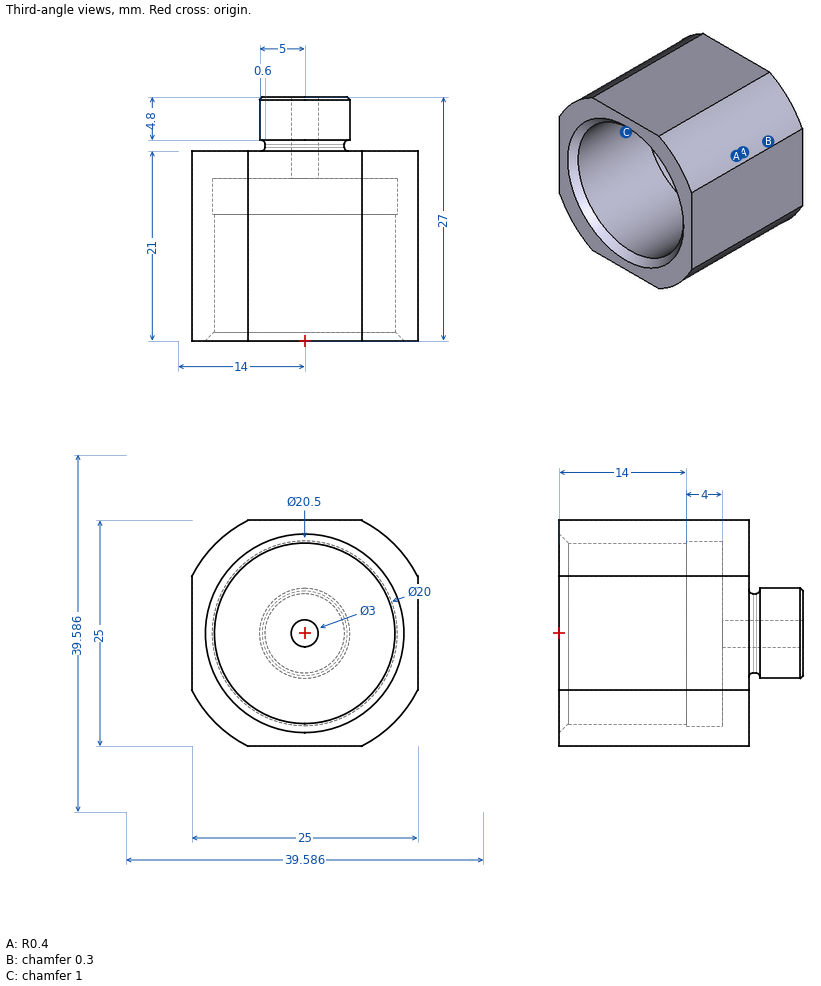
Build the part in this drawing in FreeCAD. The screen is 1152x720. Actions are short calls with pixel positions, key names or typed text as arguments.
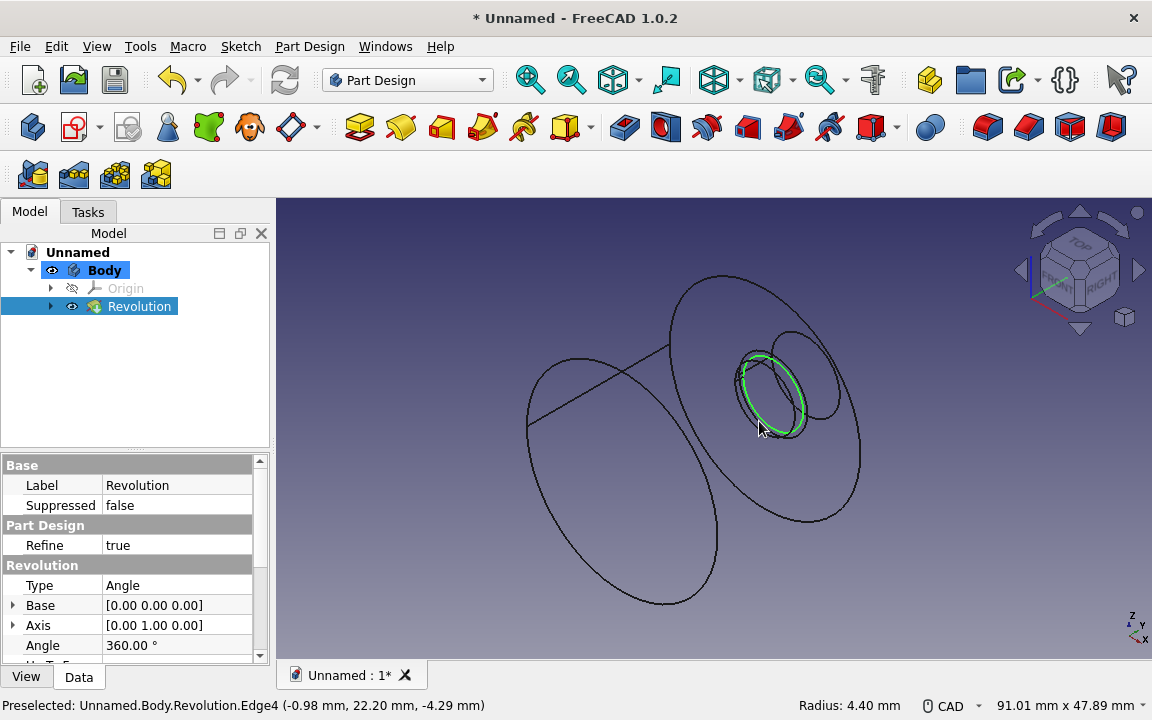
click(795, 415, ctrl)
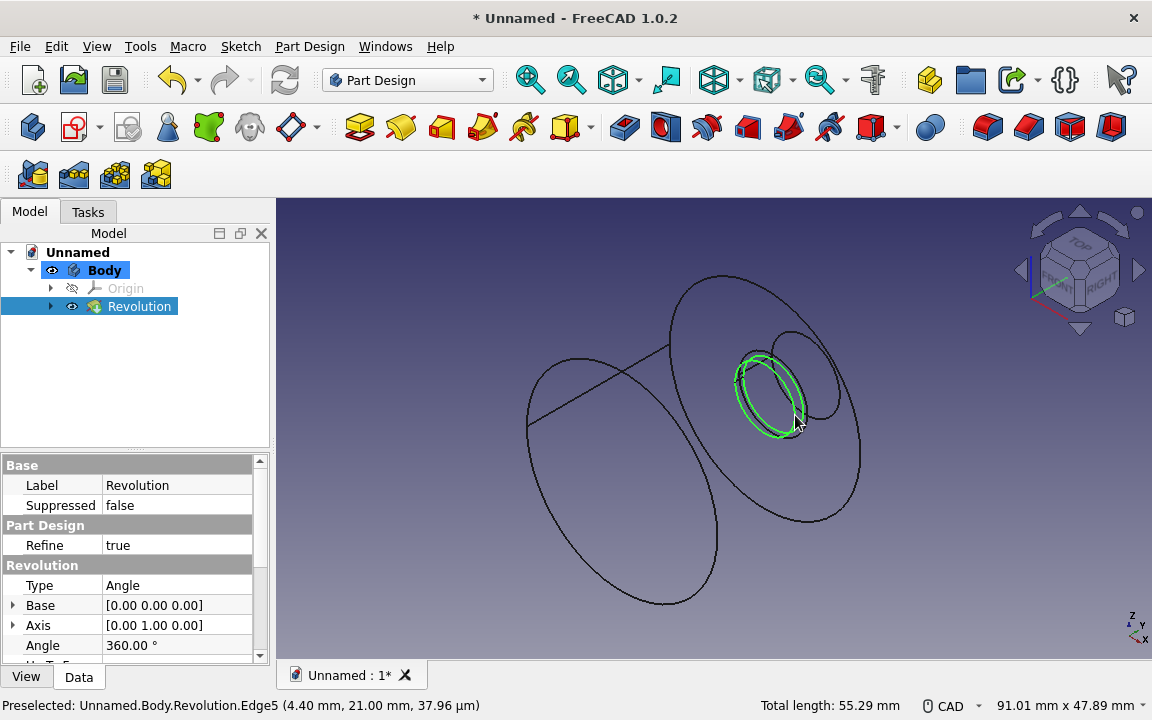
key(v)
key(1)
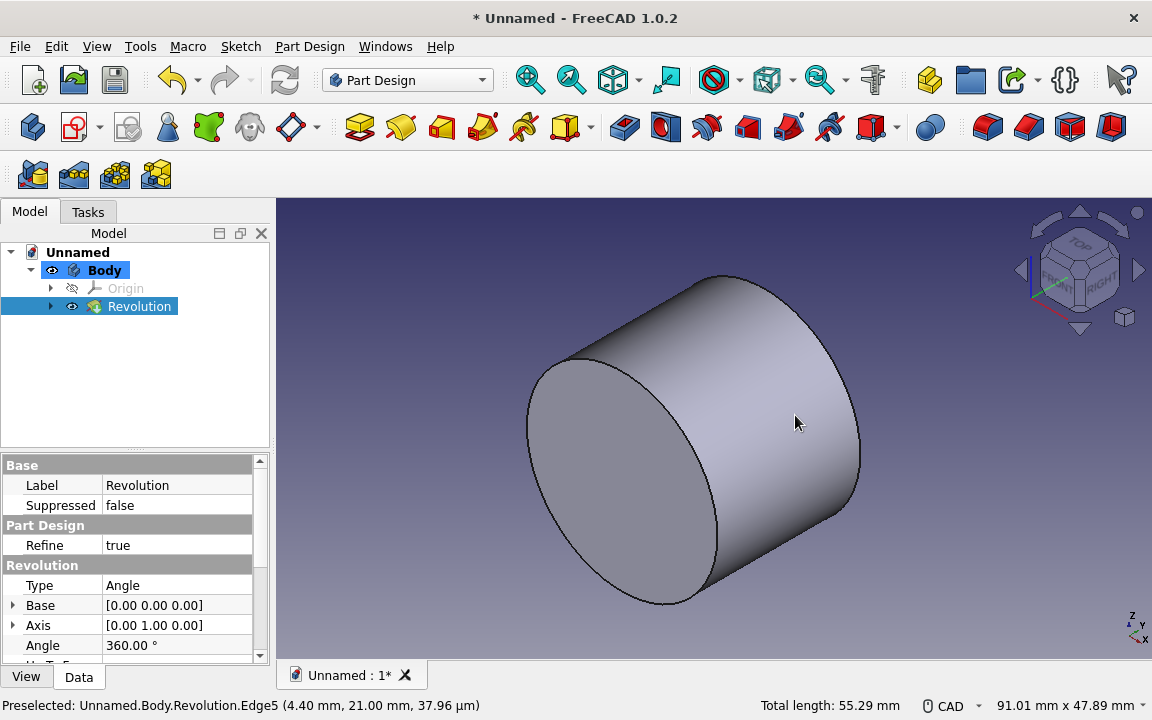
click(988, 128)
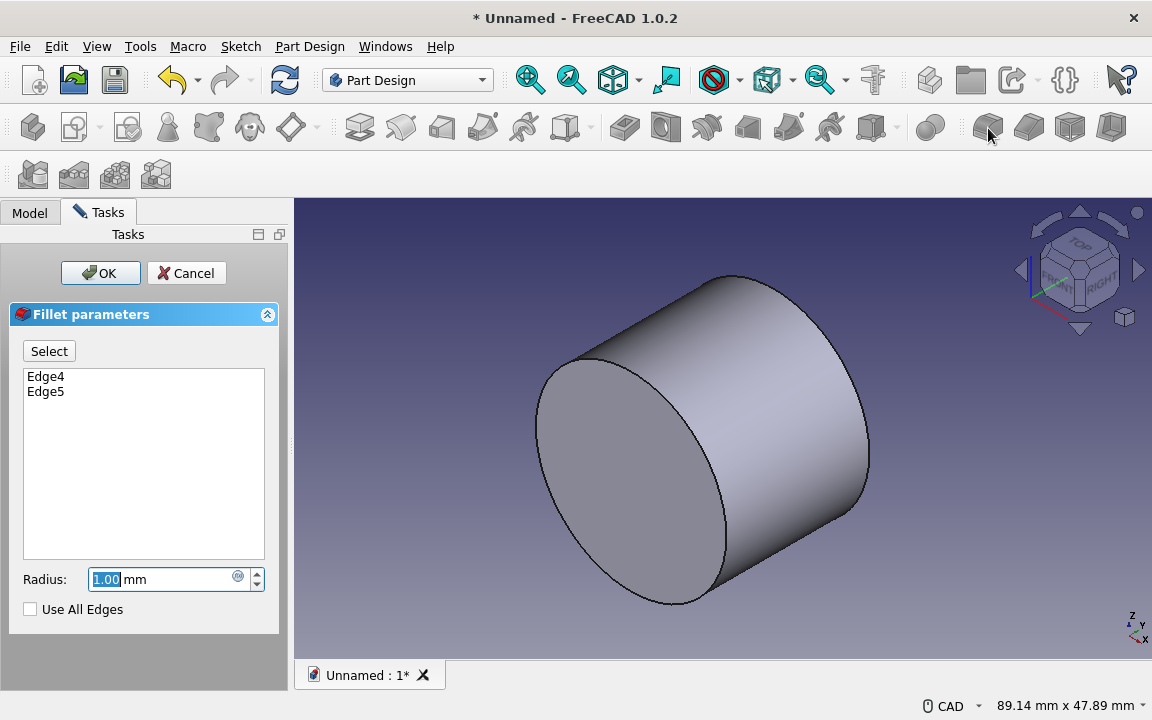
text(0.4)
key(Tab)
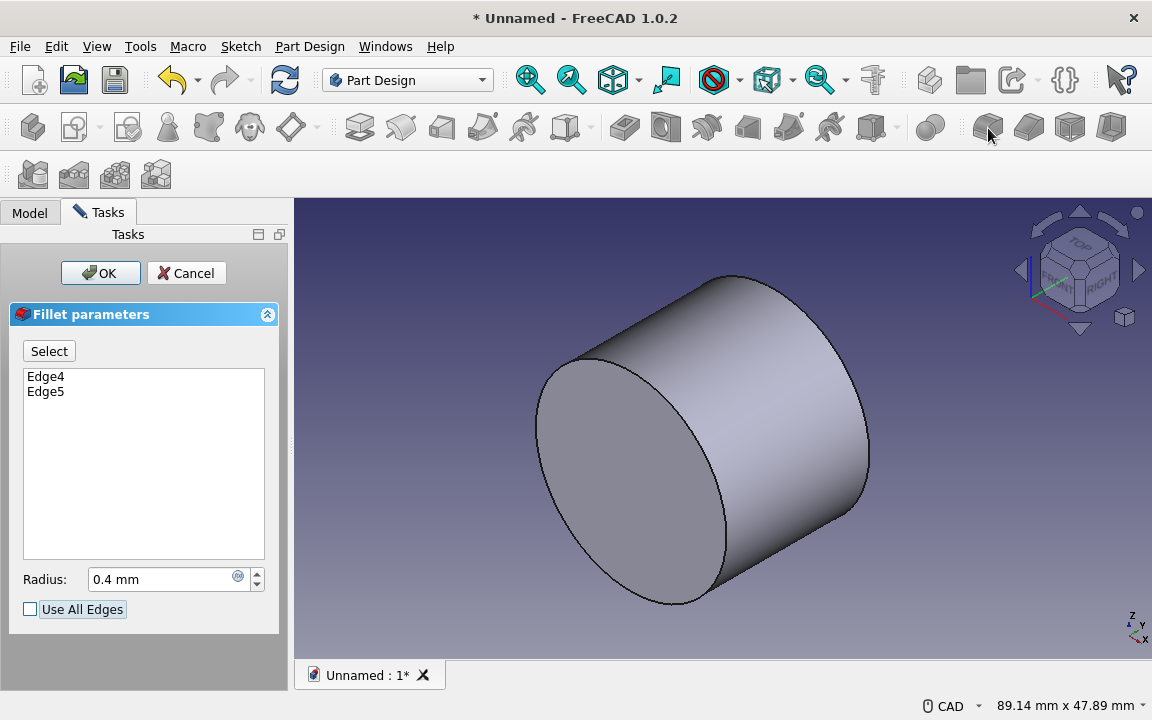
click(101, 273)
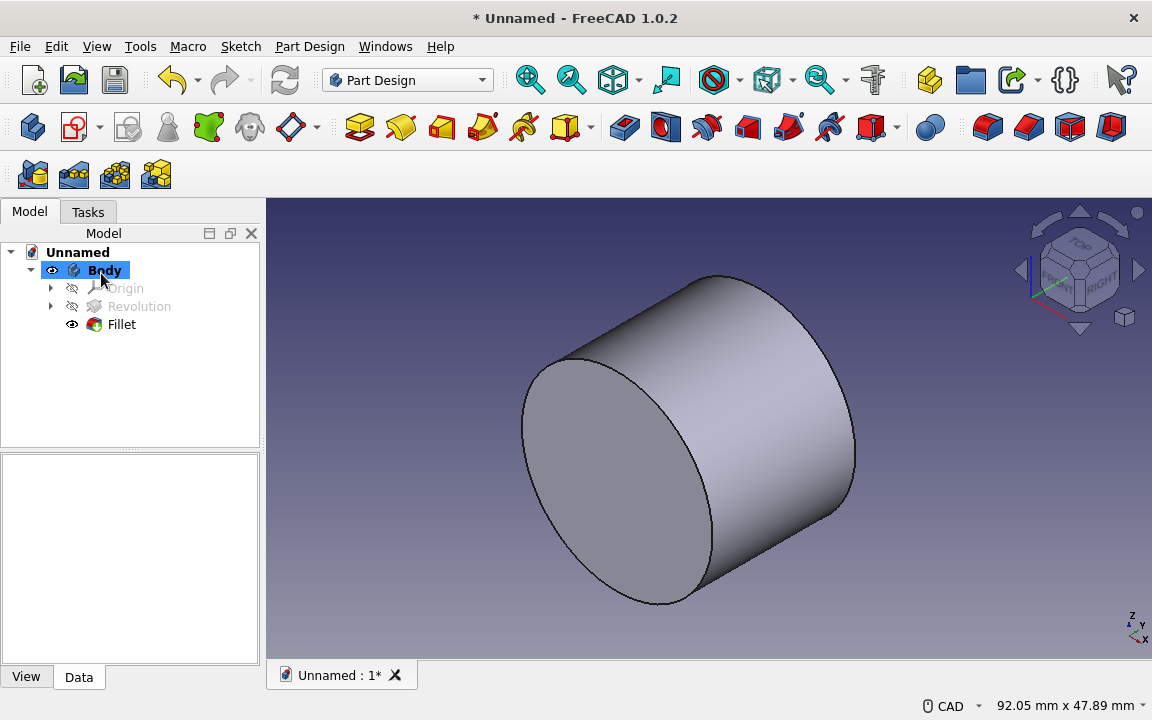
click(617, 481)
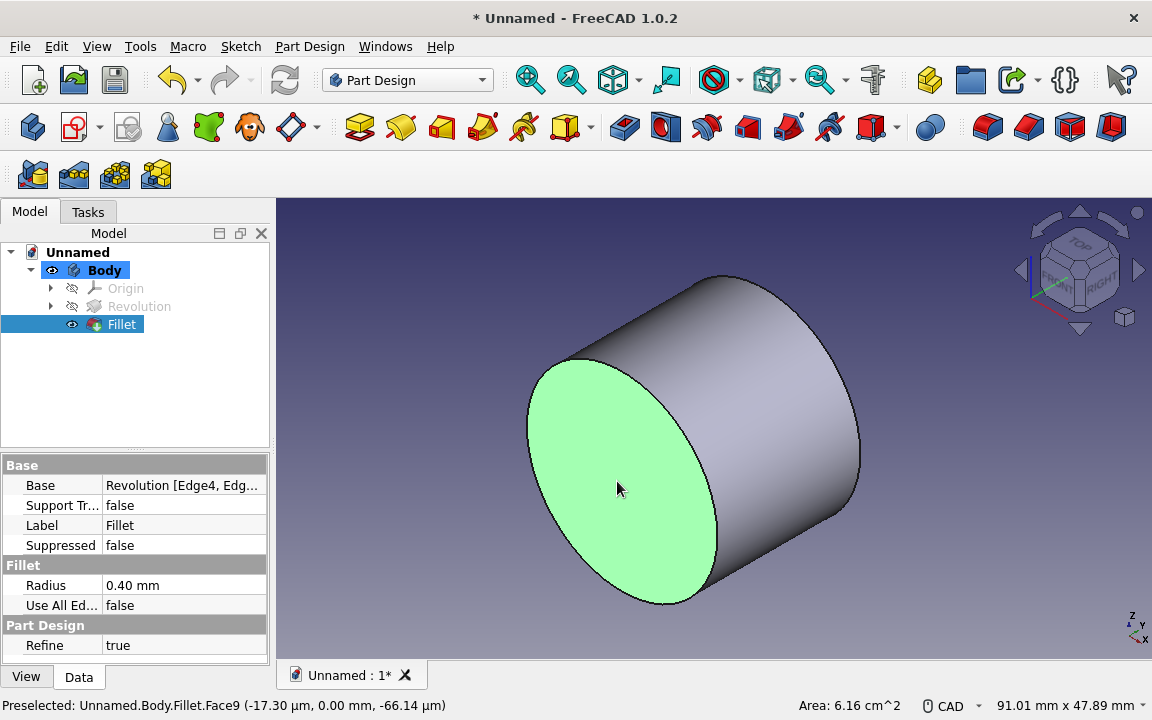
click(74, 128)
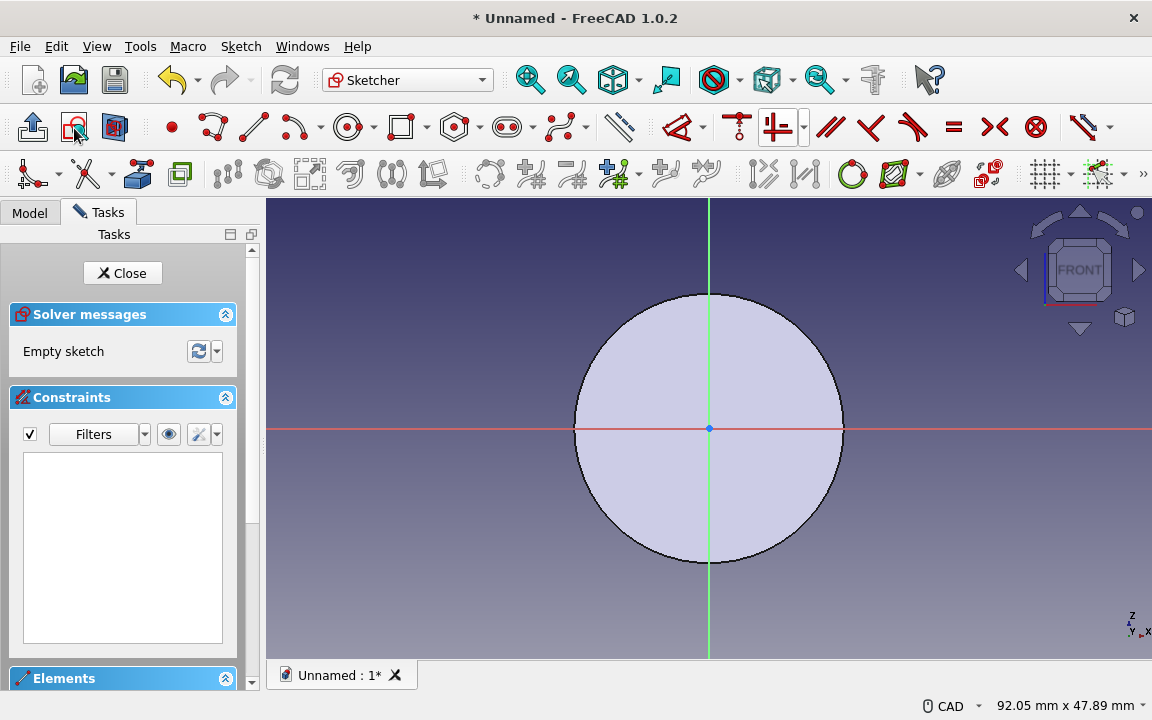
scroll(848, 428, up, 2)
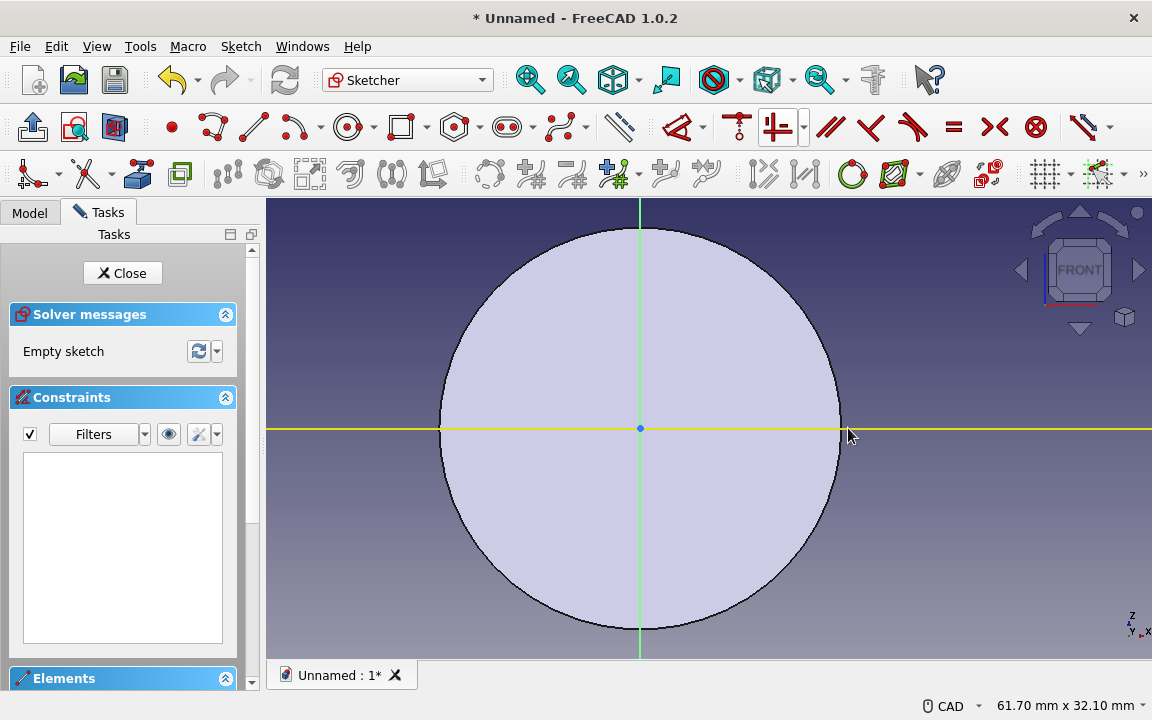
click(348, 128)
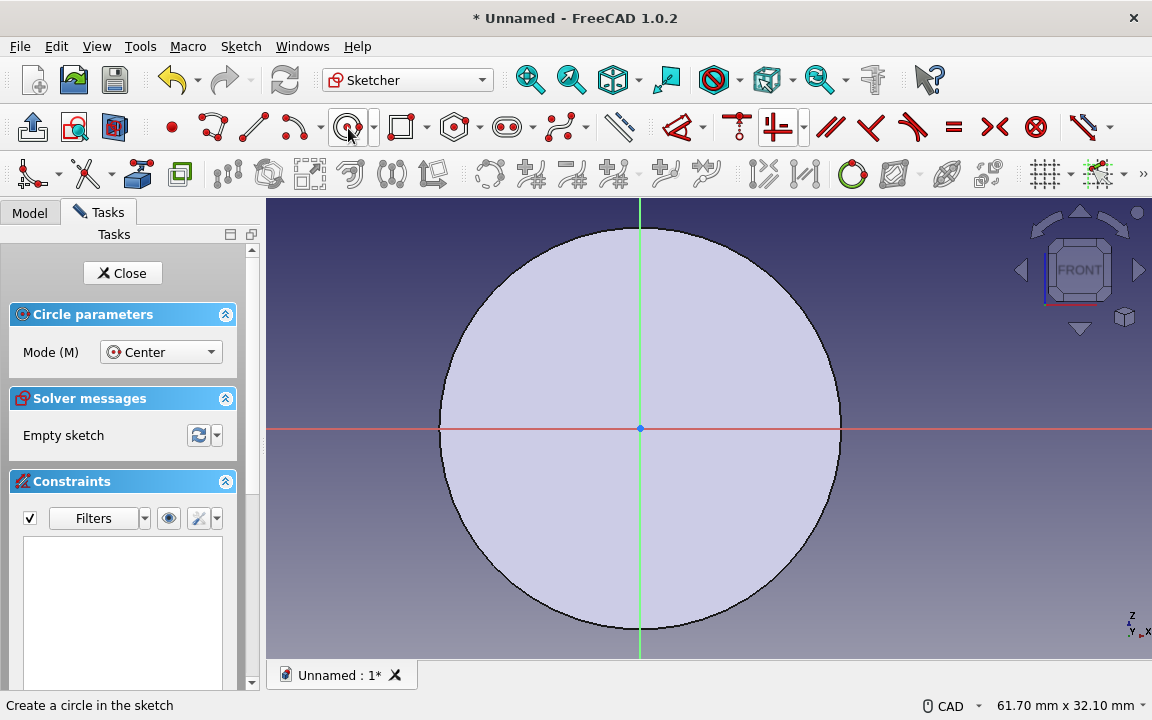
click(640, 428)
click(742, 327)
key(Escape)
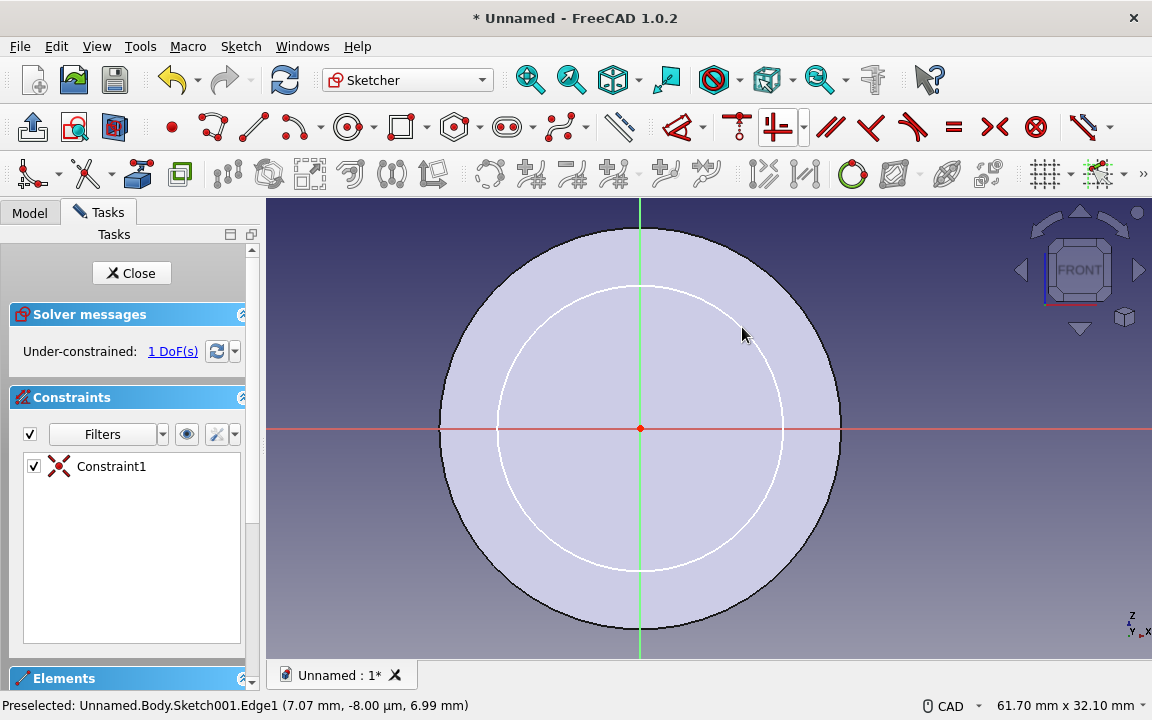
click(676, 128)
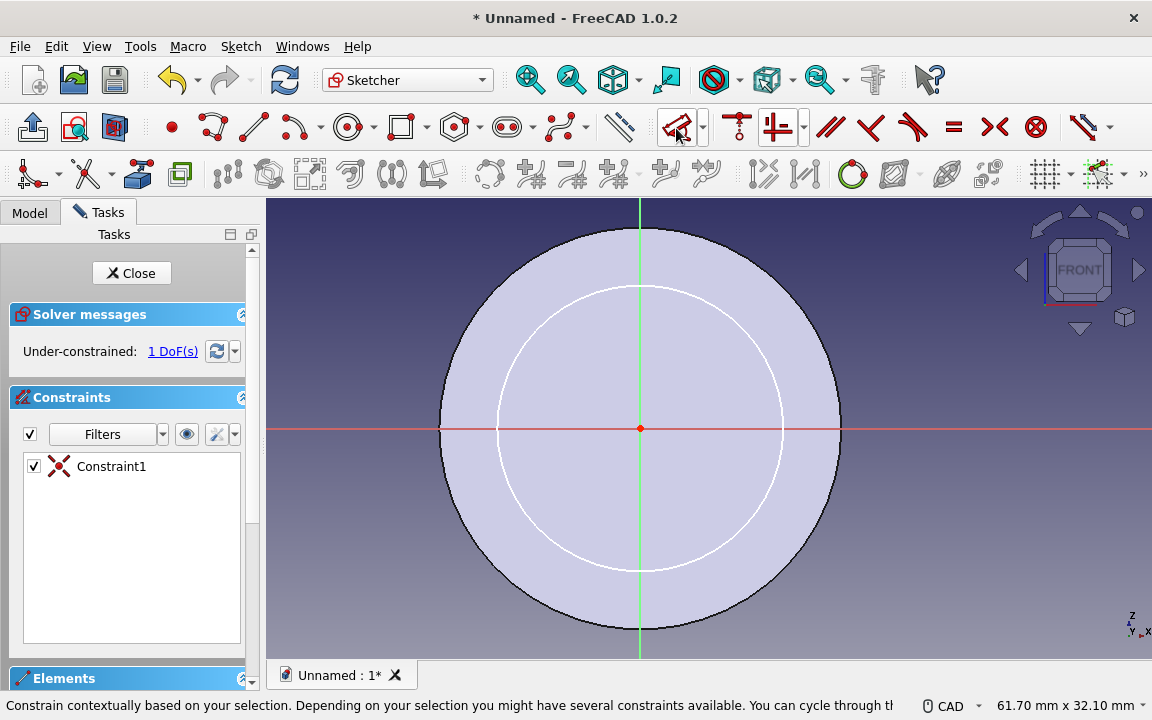
click(741, 327)
click(764, 304)